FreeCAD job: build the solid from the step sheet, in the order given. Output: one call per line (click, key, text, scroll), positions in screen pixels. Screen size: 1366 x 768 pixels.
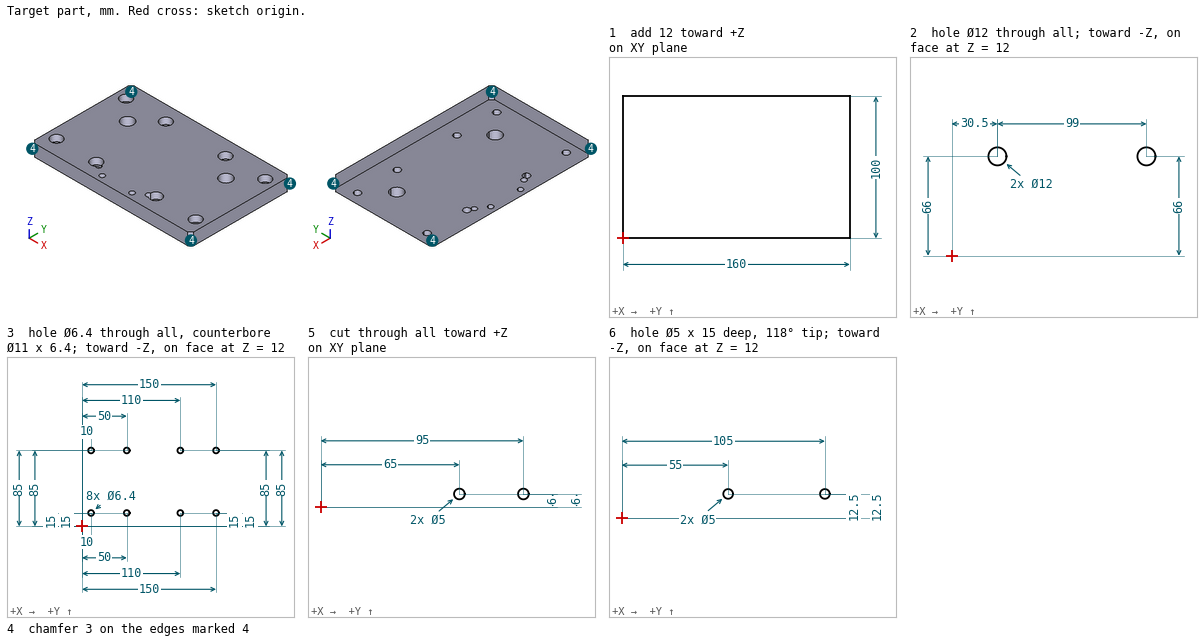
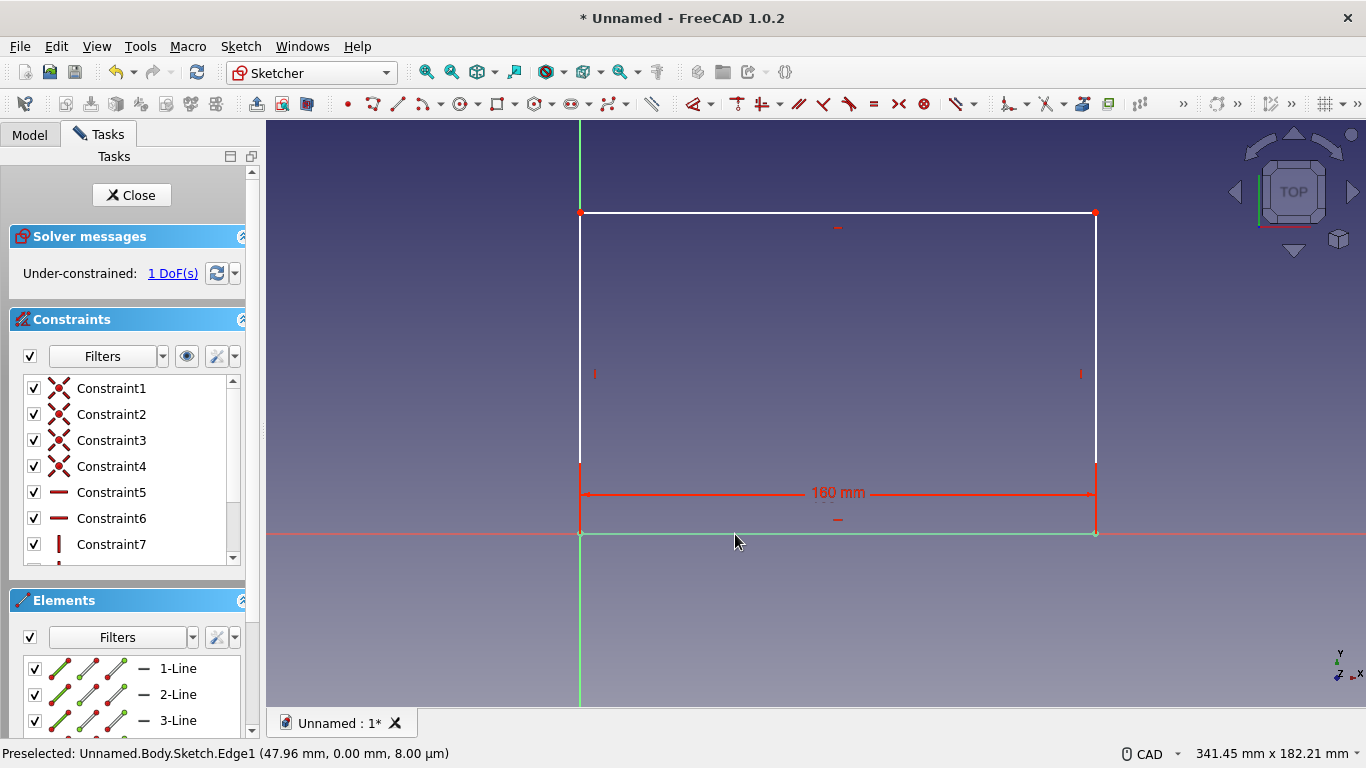
click(1096, 438)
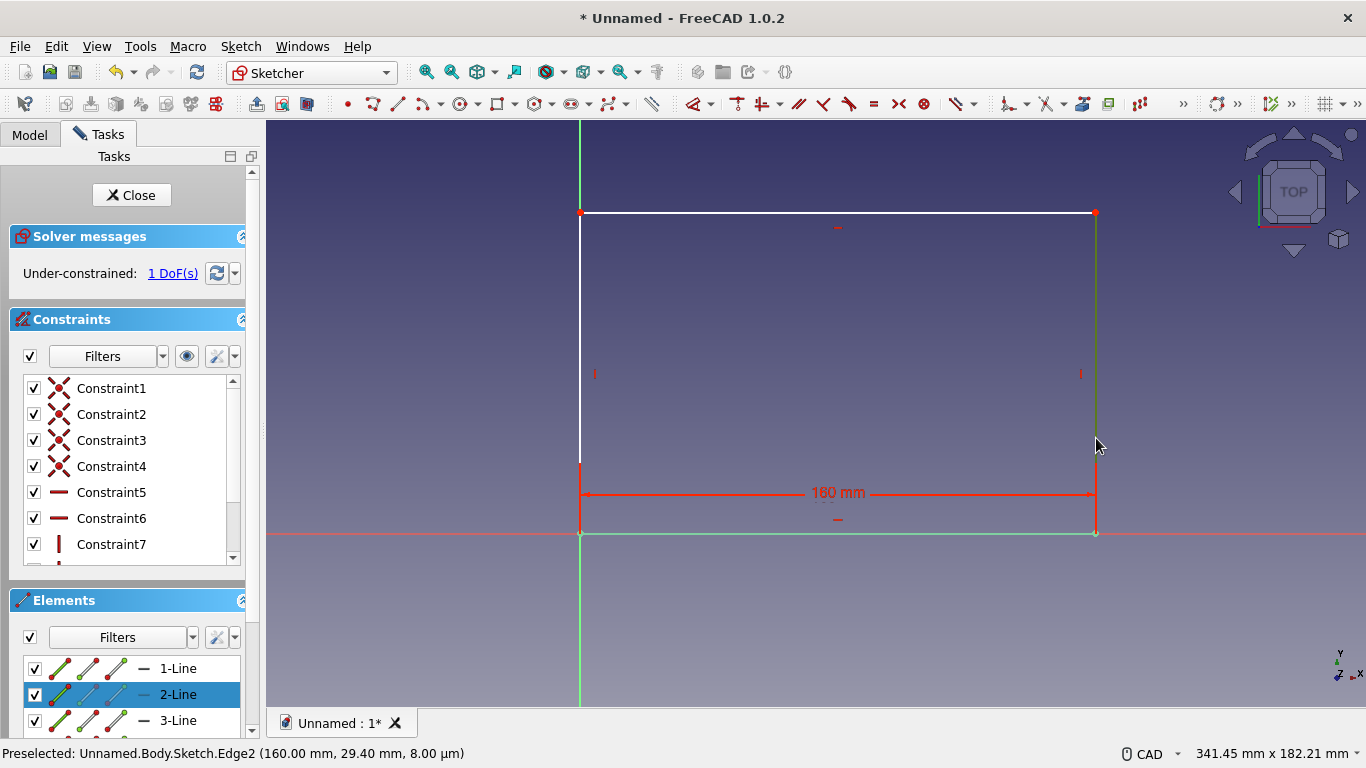
key(i)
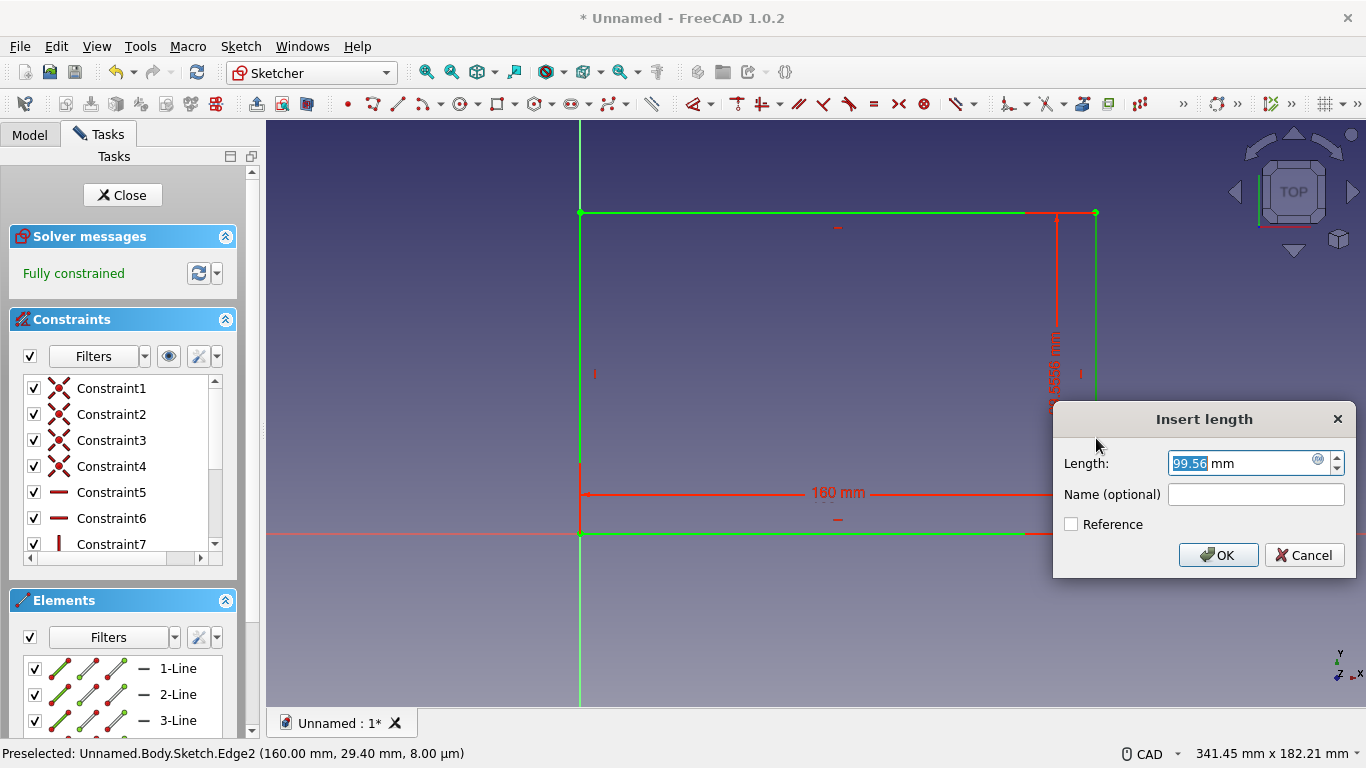
text(100)
key(Return)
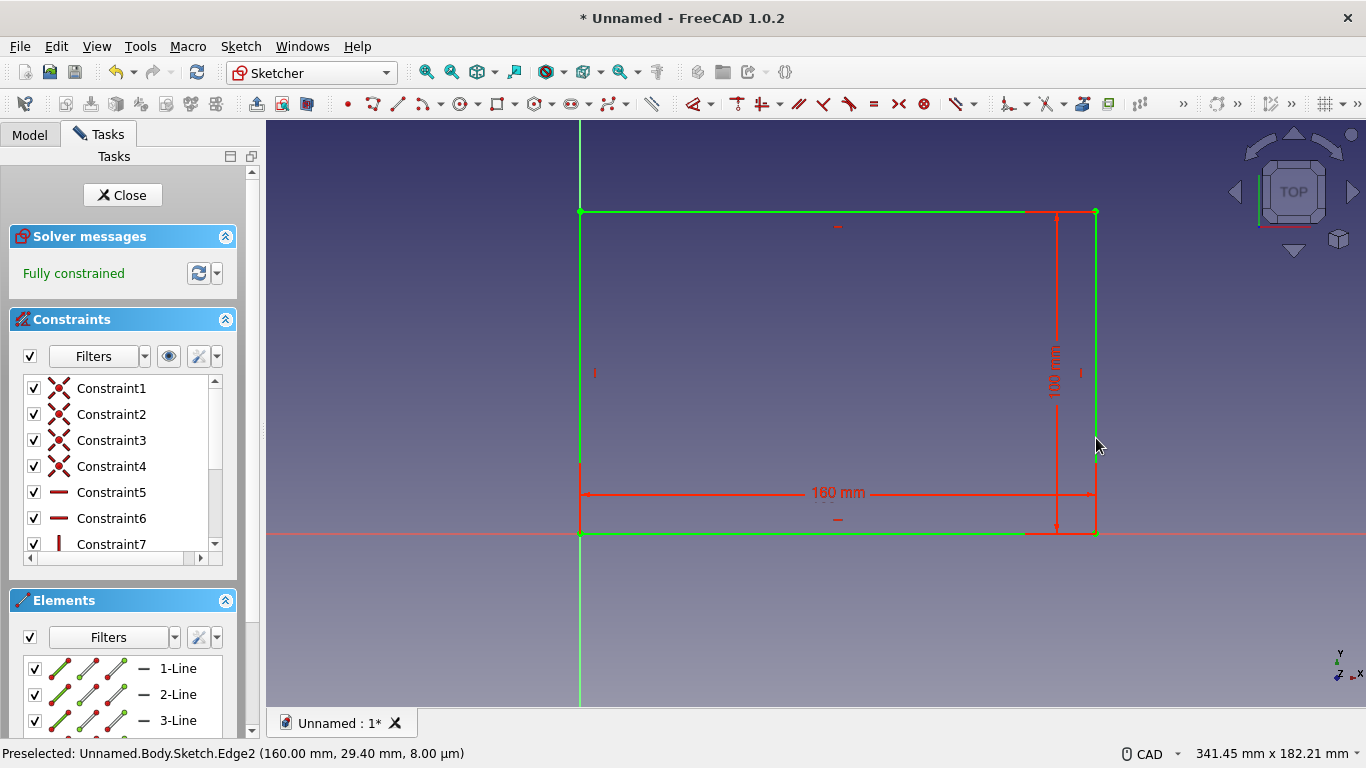
click(123, 195)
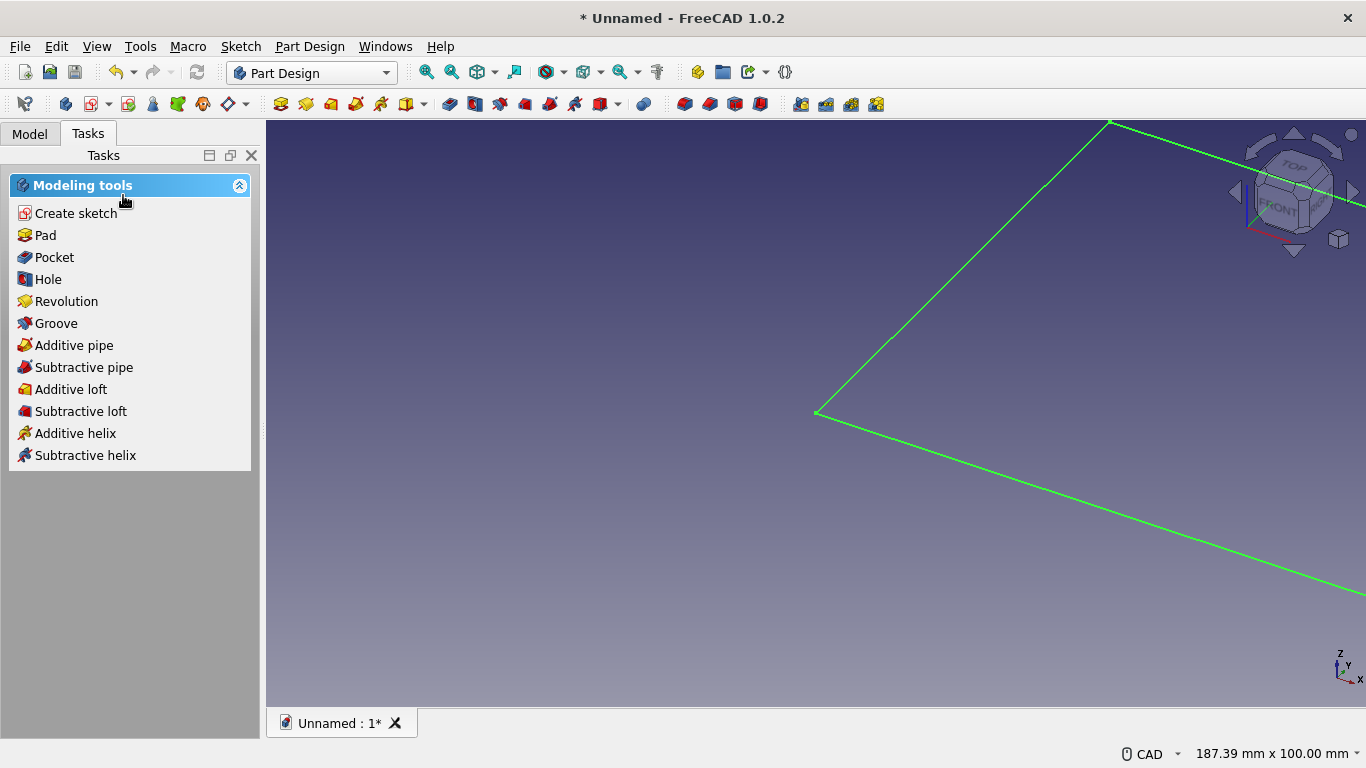
click(281, 104)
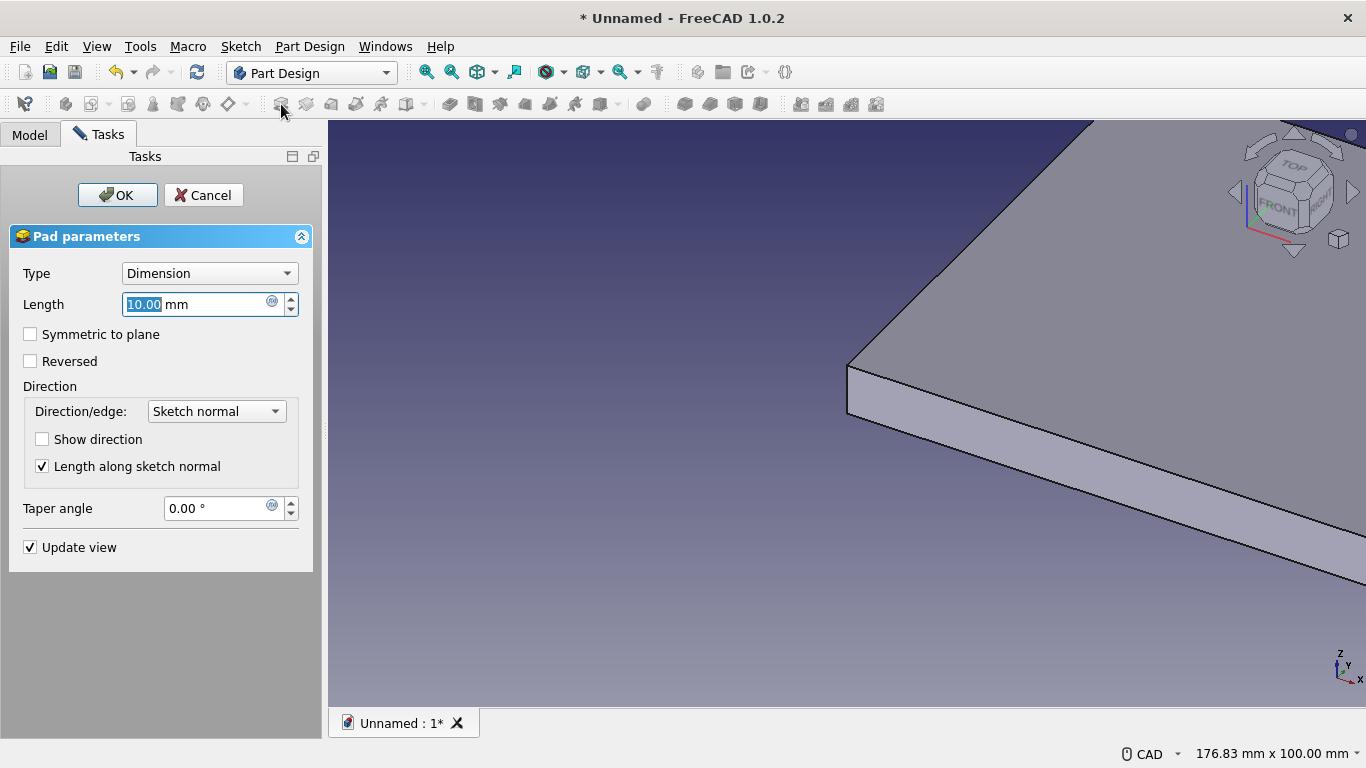
text(12)
key(Tab)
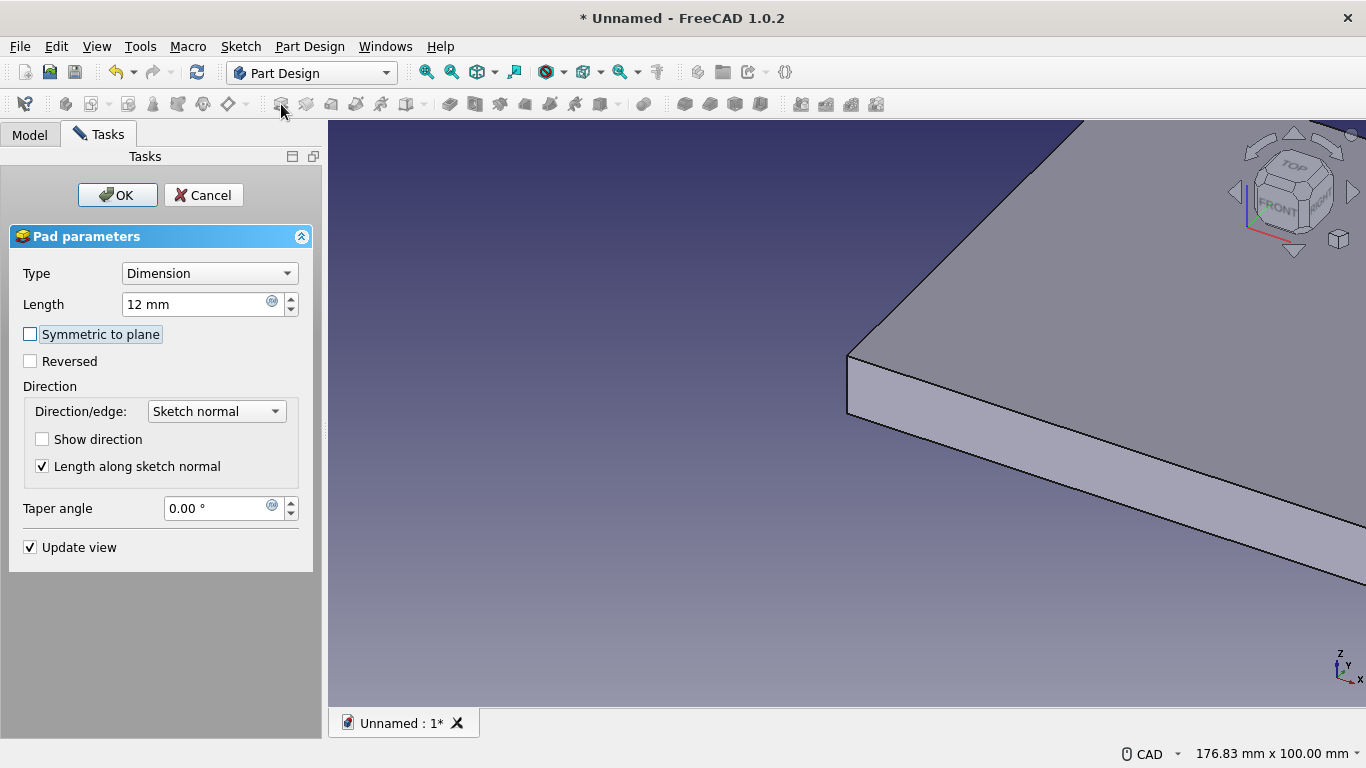
click(118, 195)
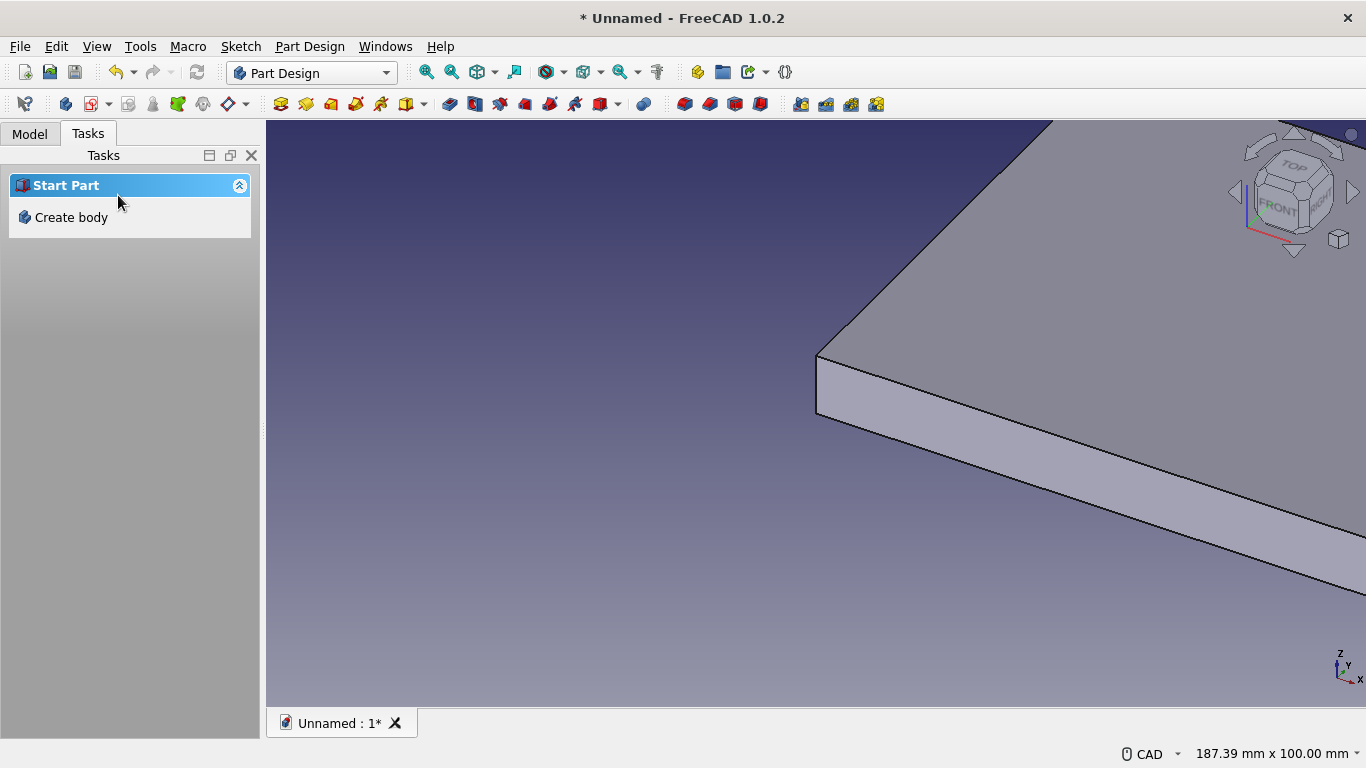
click(427, 72)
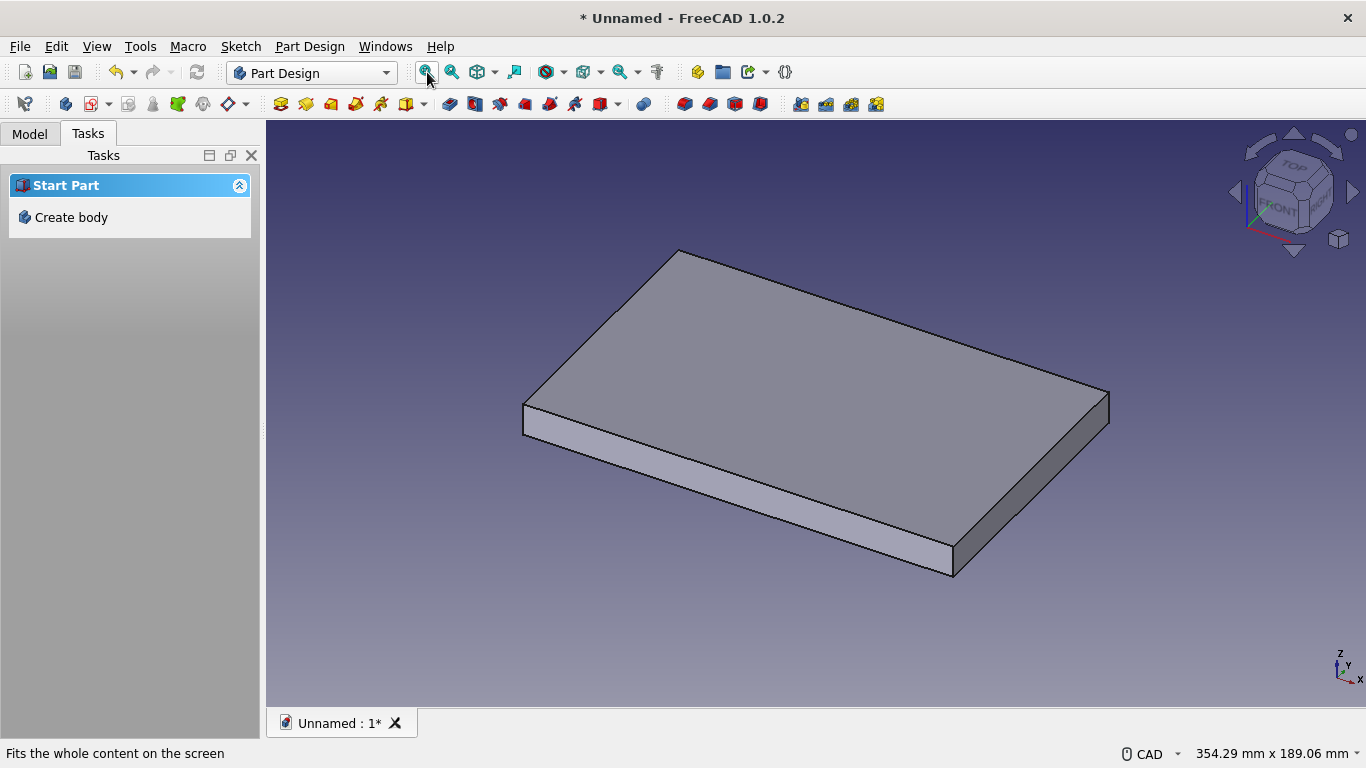
click(877, 418)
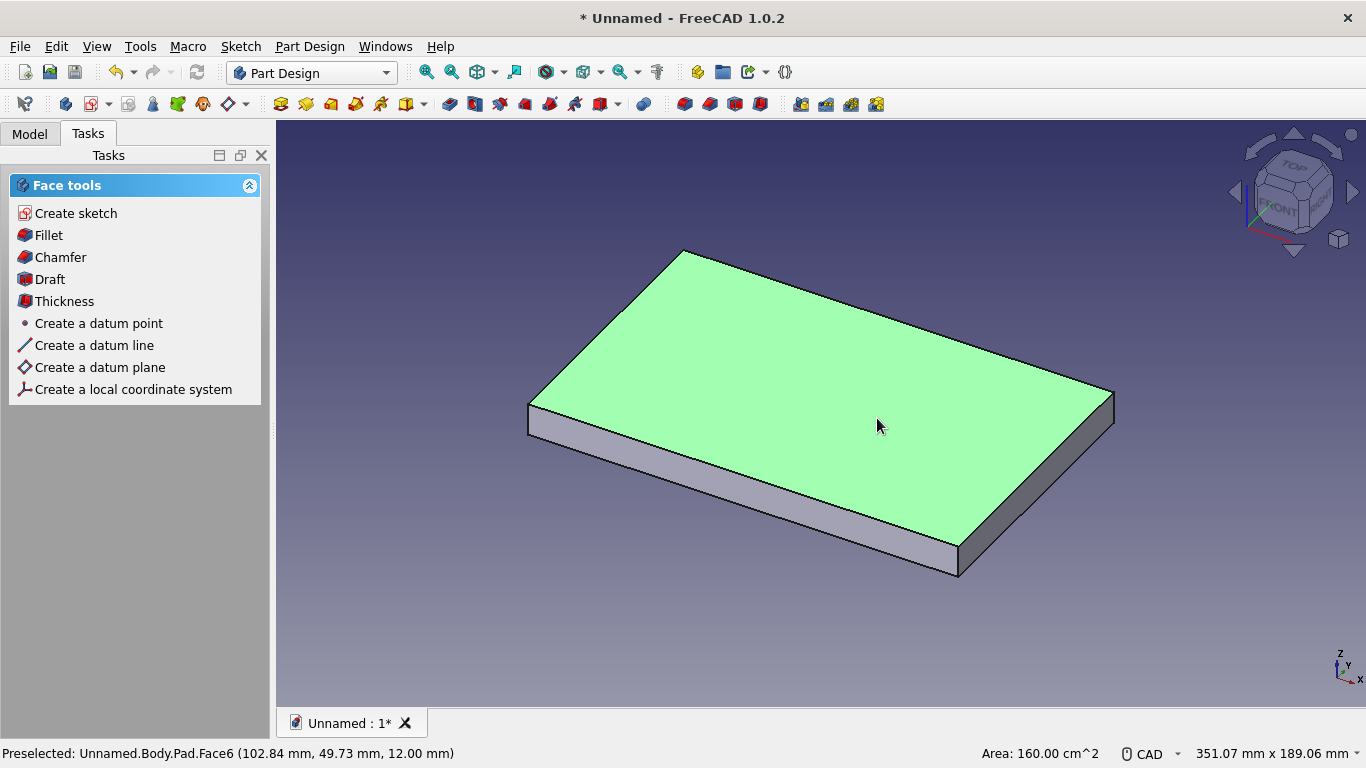
click(90, 104)